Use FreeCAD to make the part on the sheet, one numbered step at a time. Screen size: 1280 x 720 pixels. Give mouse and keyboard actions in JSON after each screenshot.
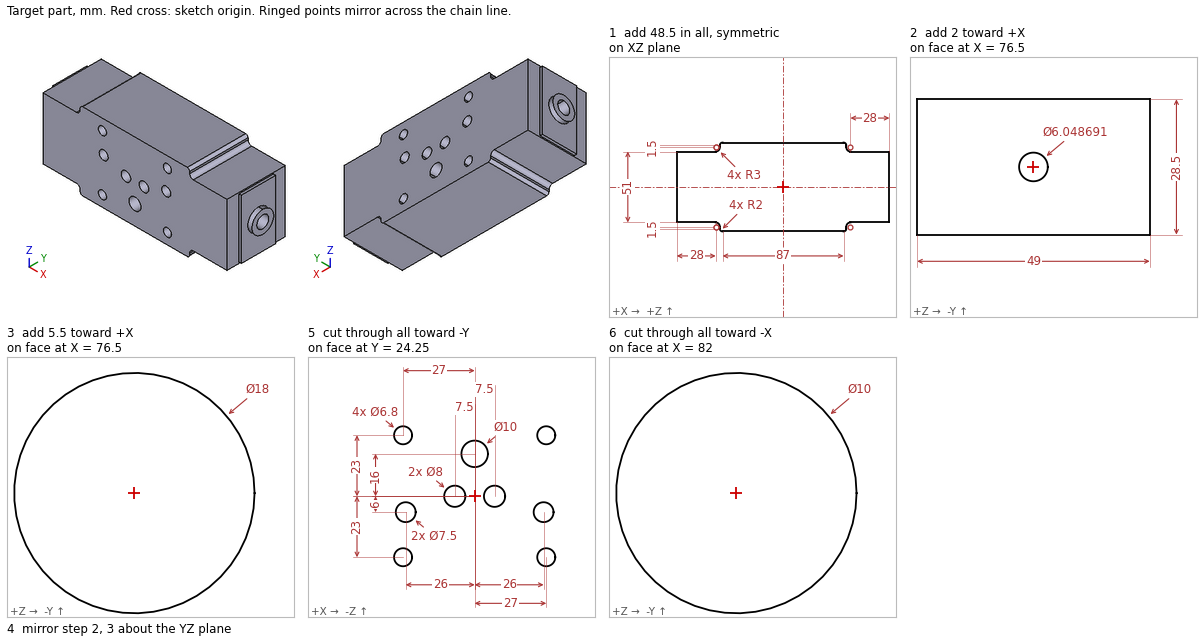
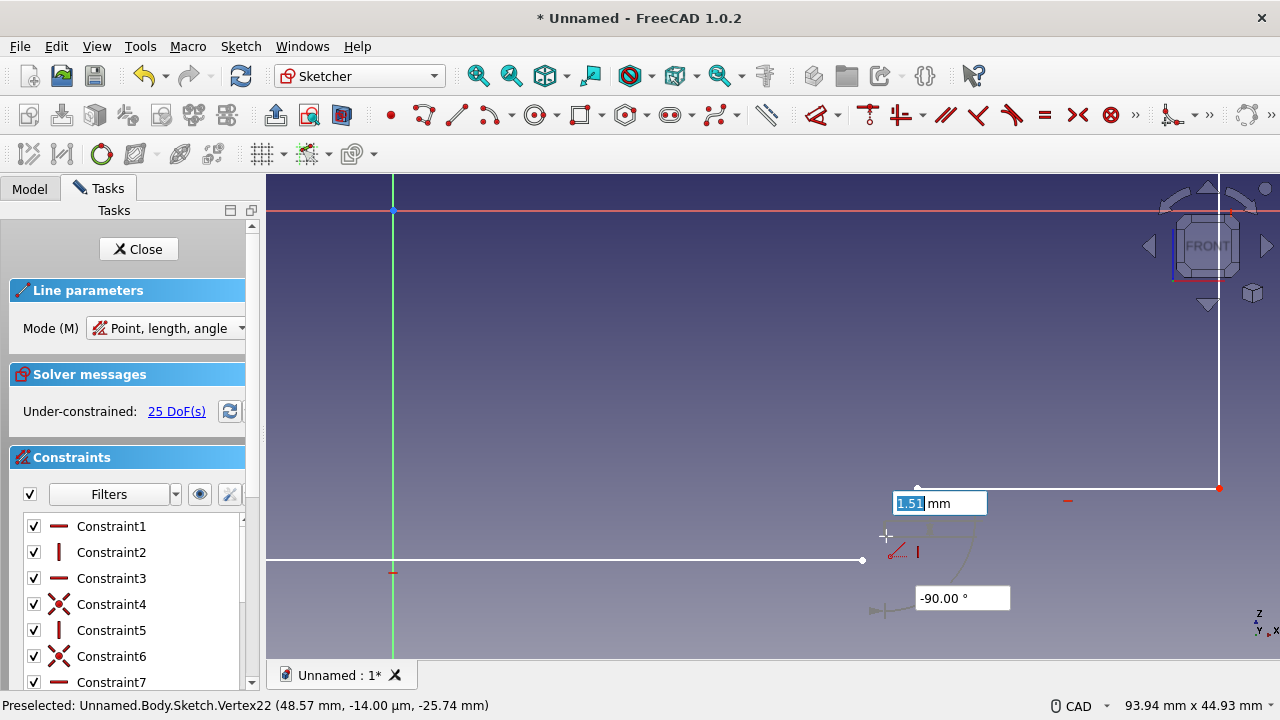
{"action": "left_click", "coordinate": [885, 535]}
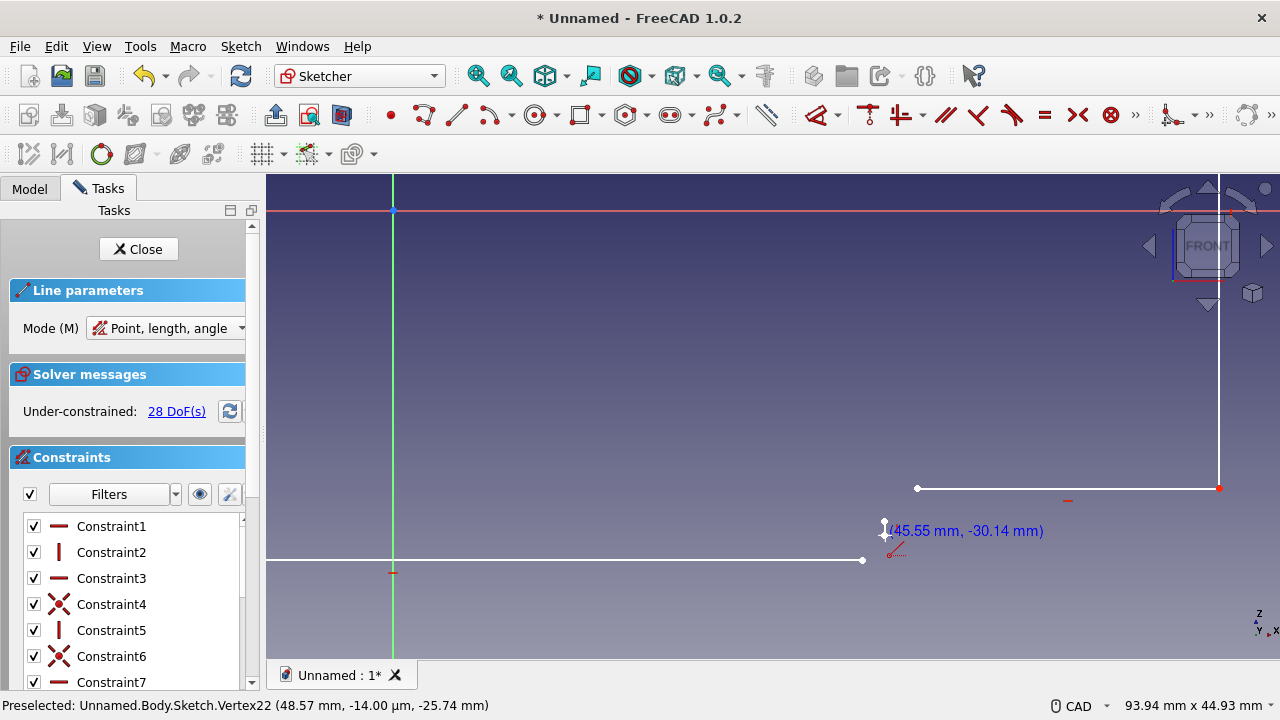
{"action": "key", "text": "g 3 a"}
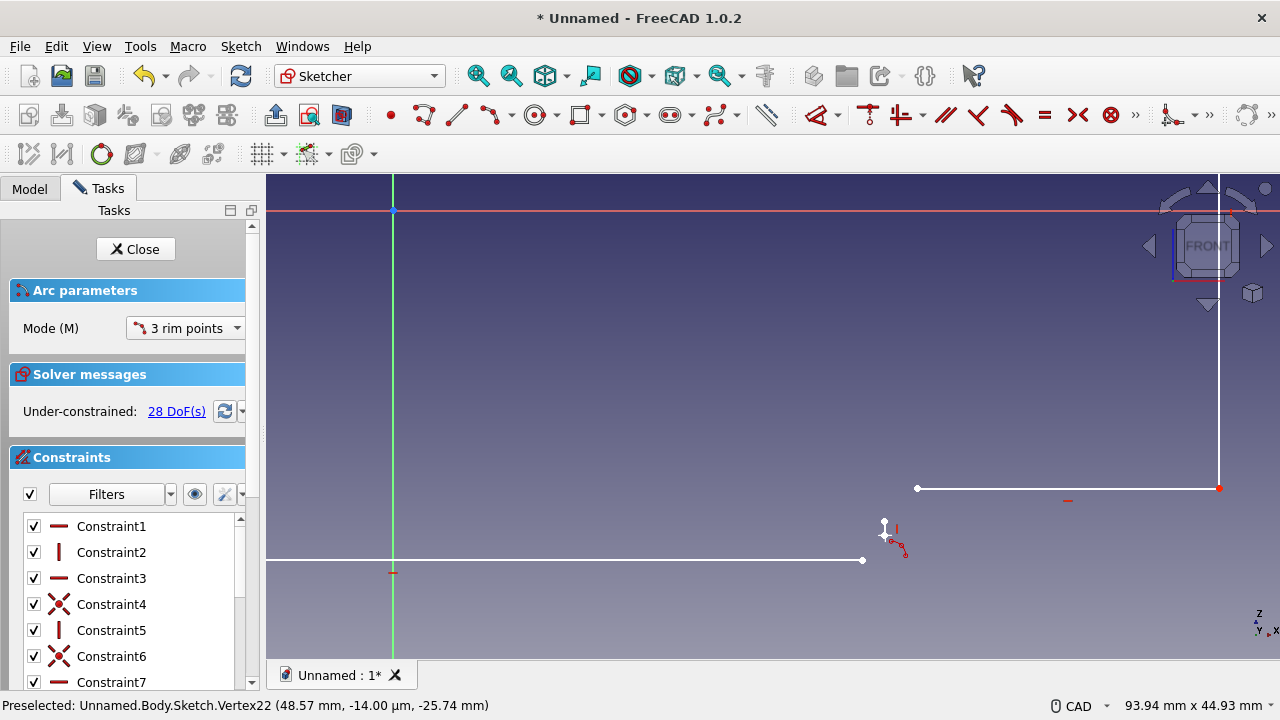
{"action": "scroll", "coordinate": [886, 536], "scroll_direction": "down", "scroll_amount": 5}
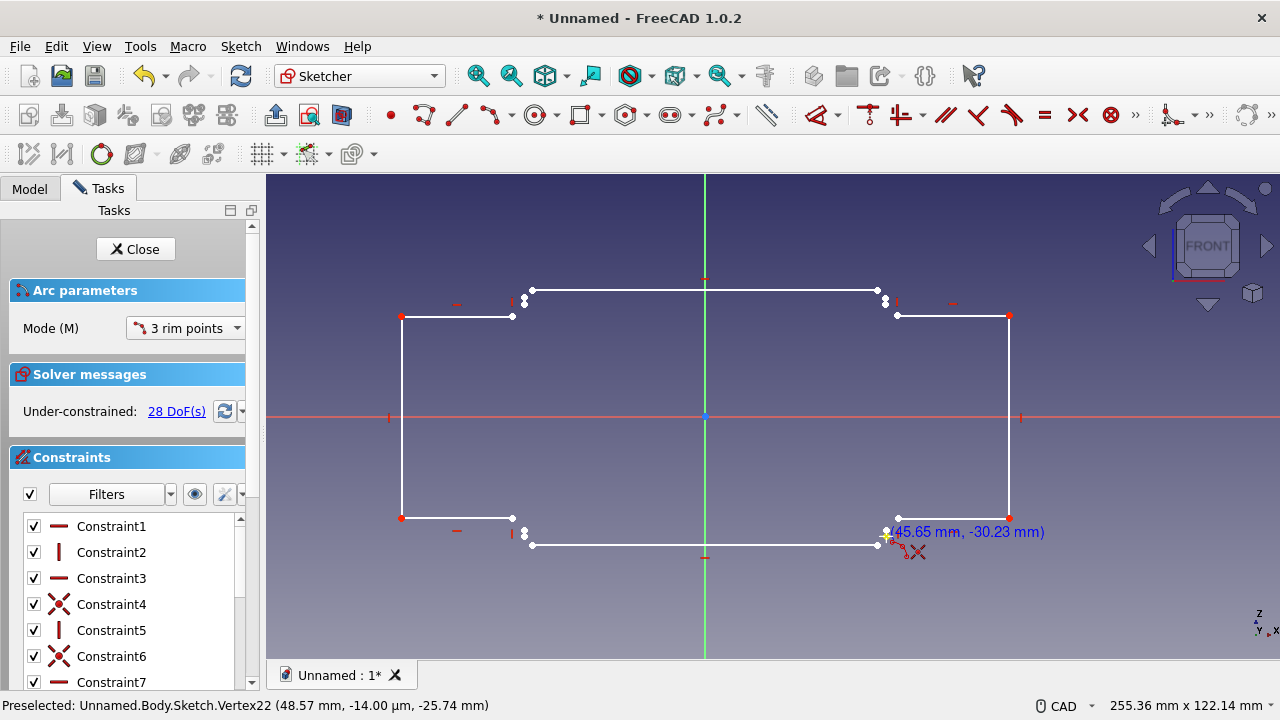
{"action": "scroll", "coordinate": [532, 544], "scroll_direction": "up", "scroll_amount": 2}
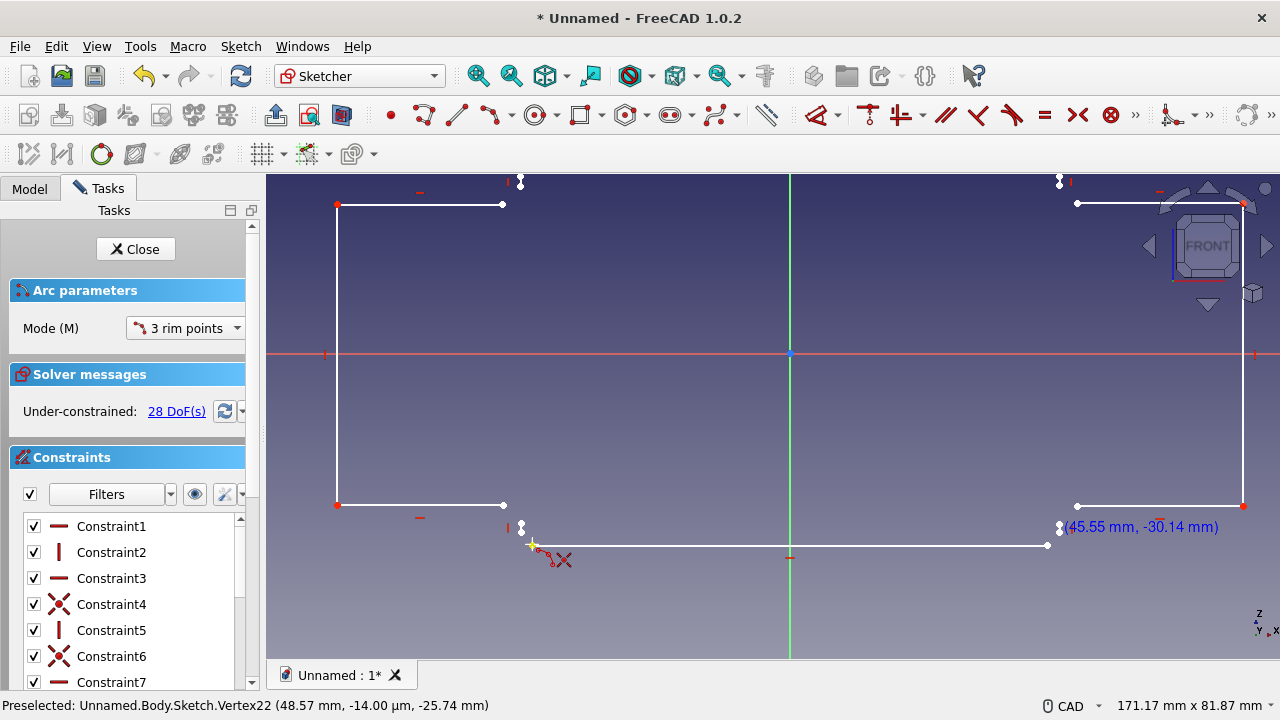
{"action": "left_click", "coordinate": [533, 546]}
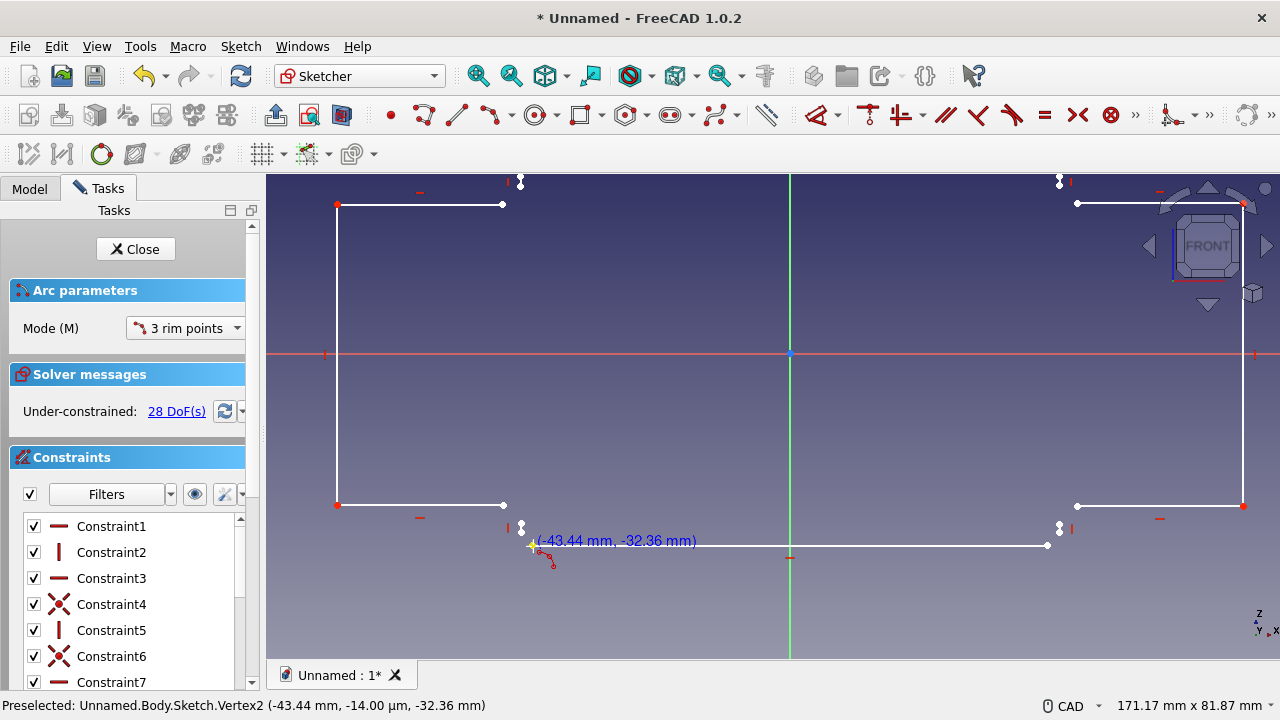
{"action": "scroll", "coordinate": [521, 532], "scroll_direction": "up", "scroll_amount": 7}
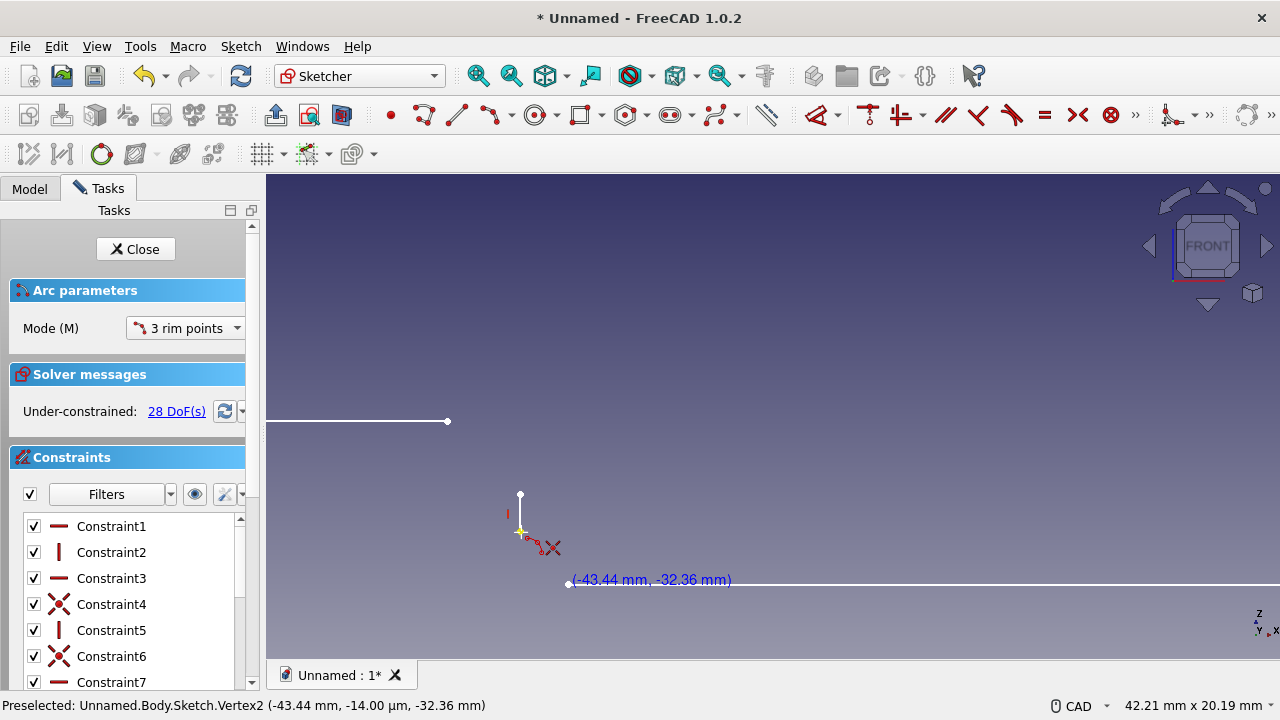
{"action": "left_click", "coordinate": [520, 532]}
{"action": "left_click", "coordinate": [533, 562]}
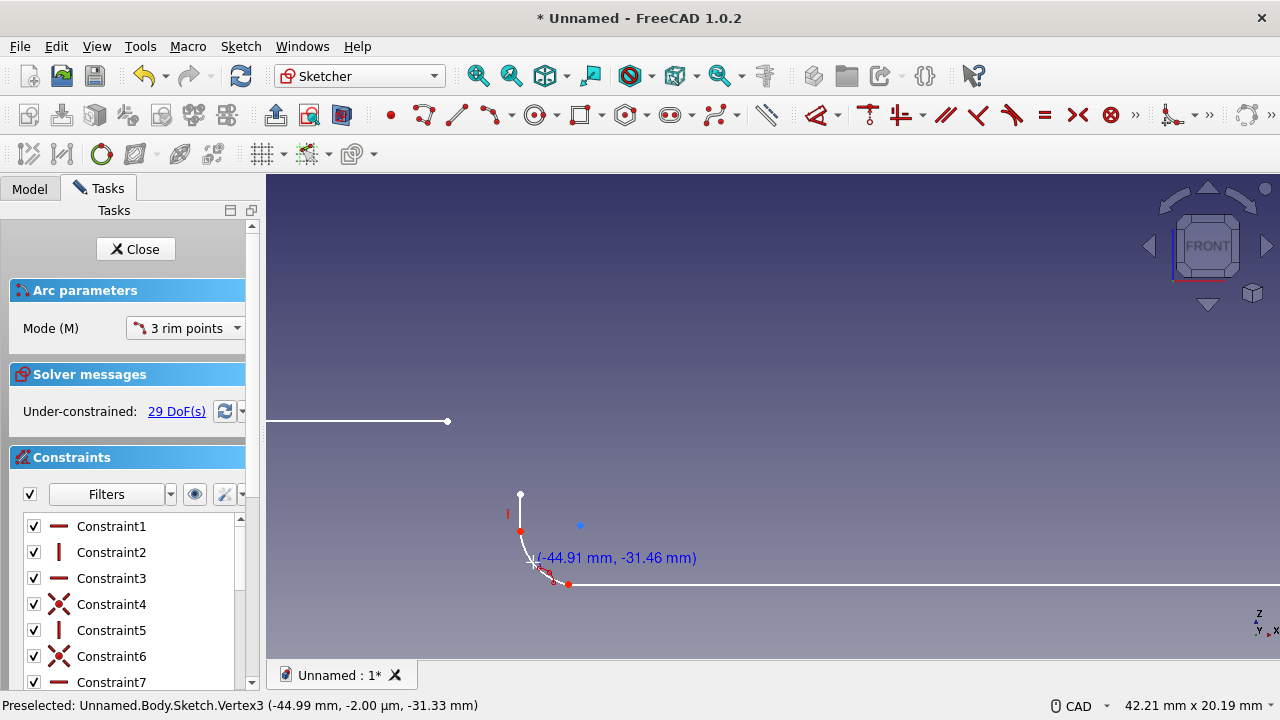
{"action": "left_click", "coordinate": [520, 495]}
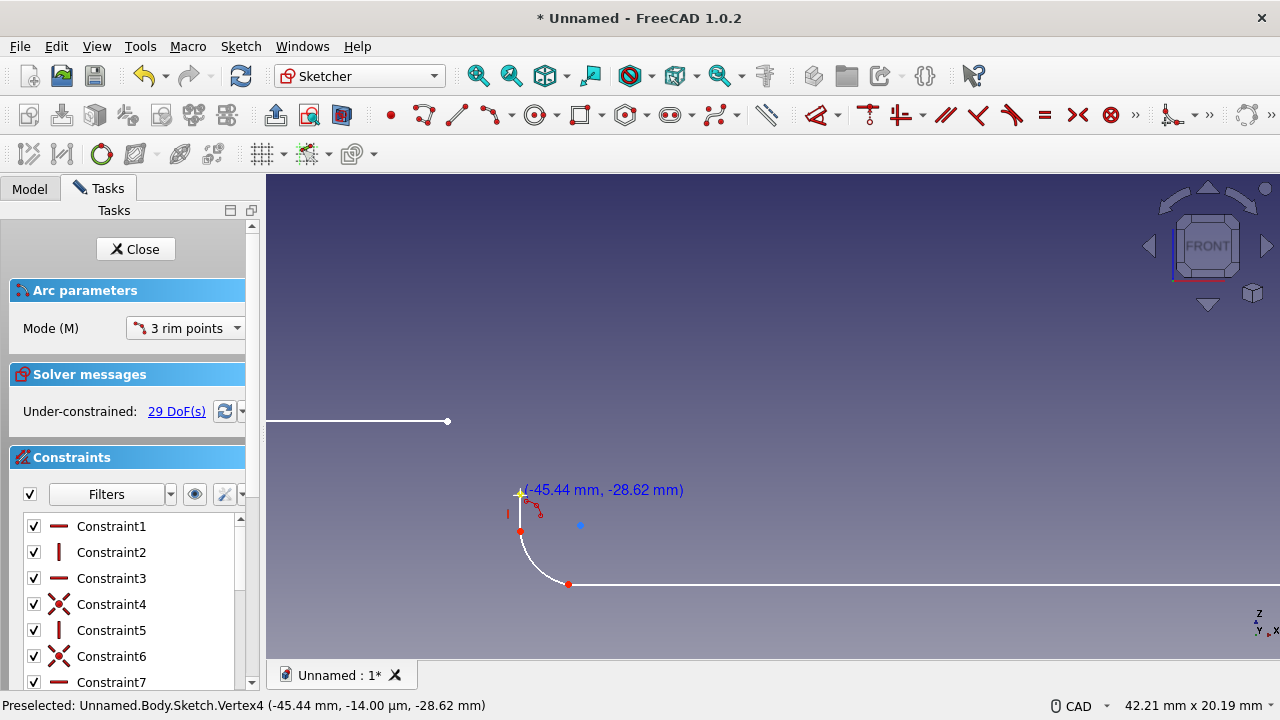
{"action": "scroll", "coordinate": [525, 537], "scroll_direction": "down", "scroll_amount": 9}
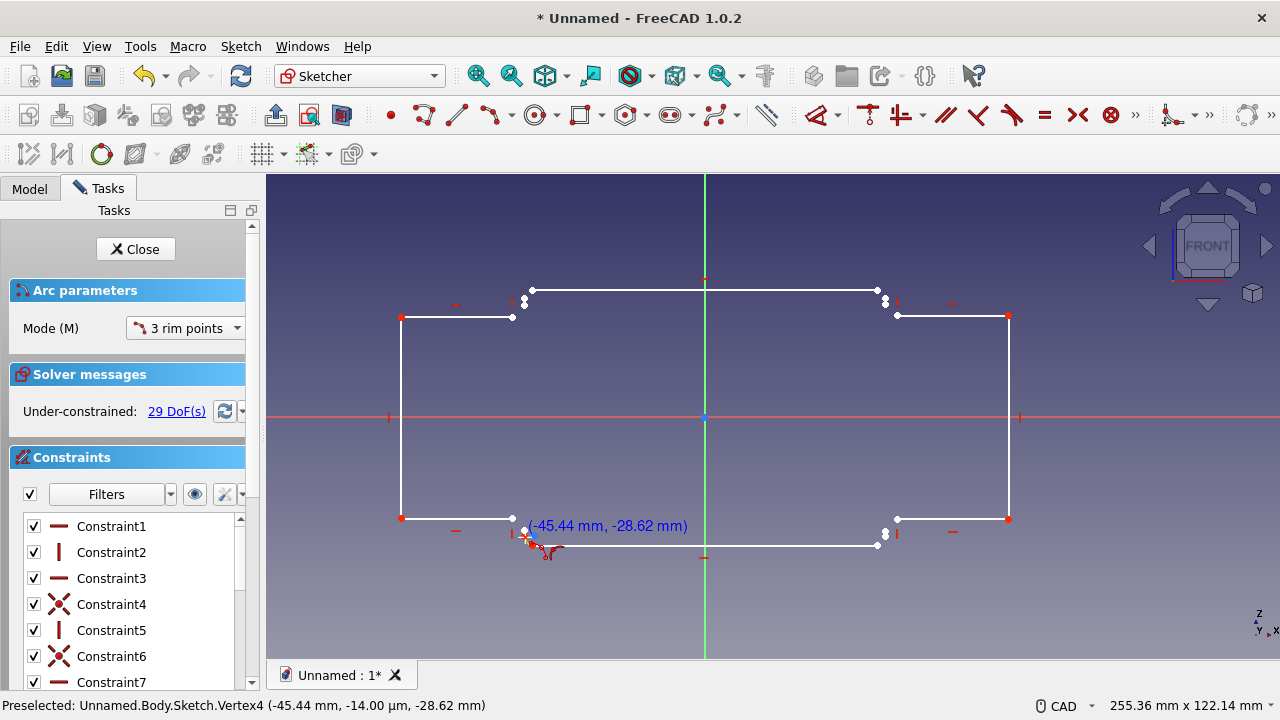
{"action": "left_click", "coordinate": [512, 519]}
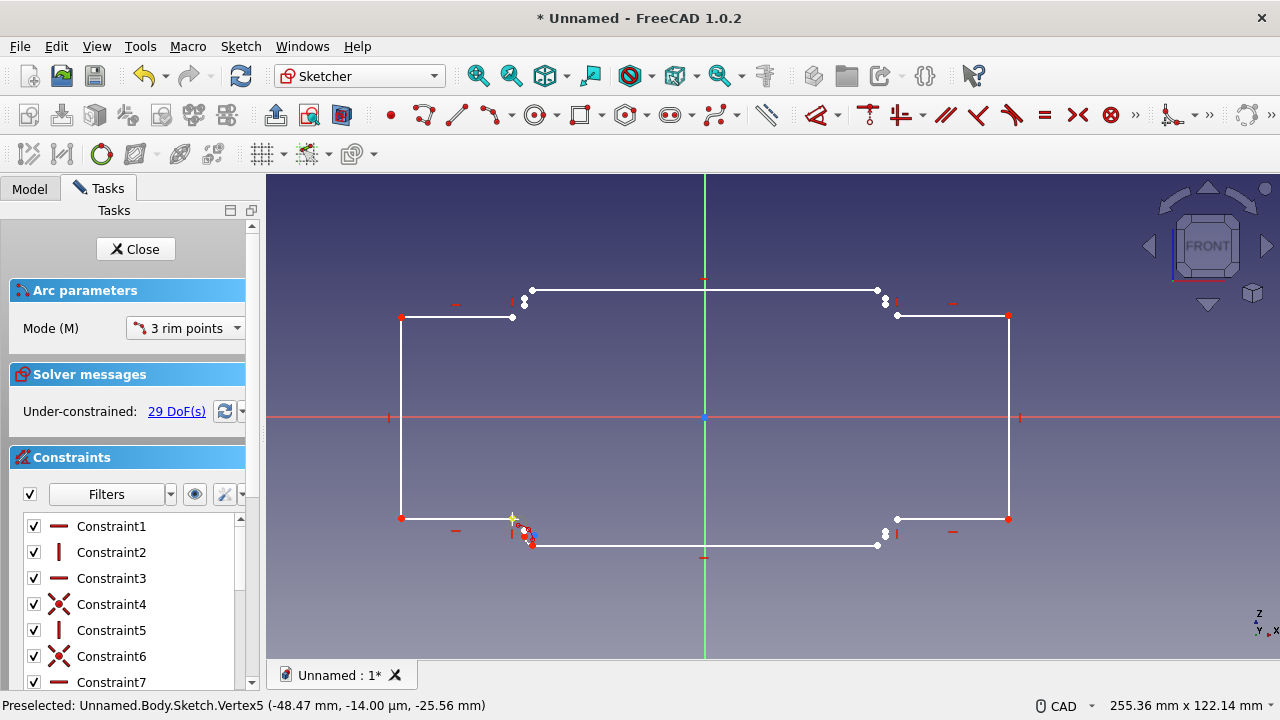
{"action": "scroll", "coordinate": [521, 522], "scroll_direction": "up", "scroll_amount": 8}